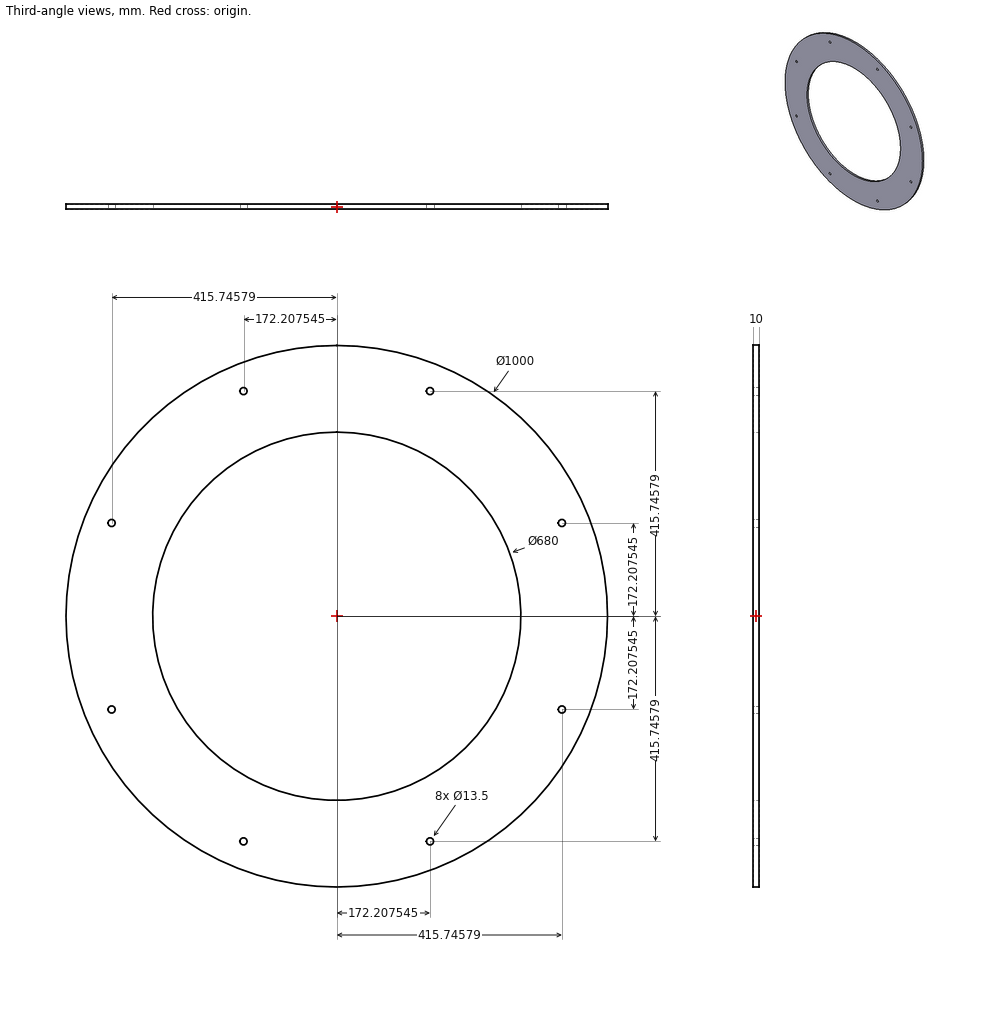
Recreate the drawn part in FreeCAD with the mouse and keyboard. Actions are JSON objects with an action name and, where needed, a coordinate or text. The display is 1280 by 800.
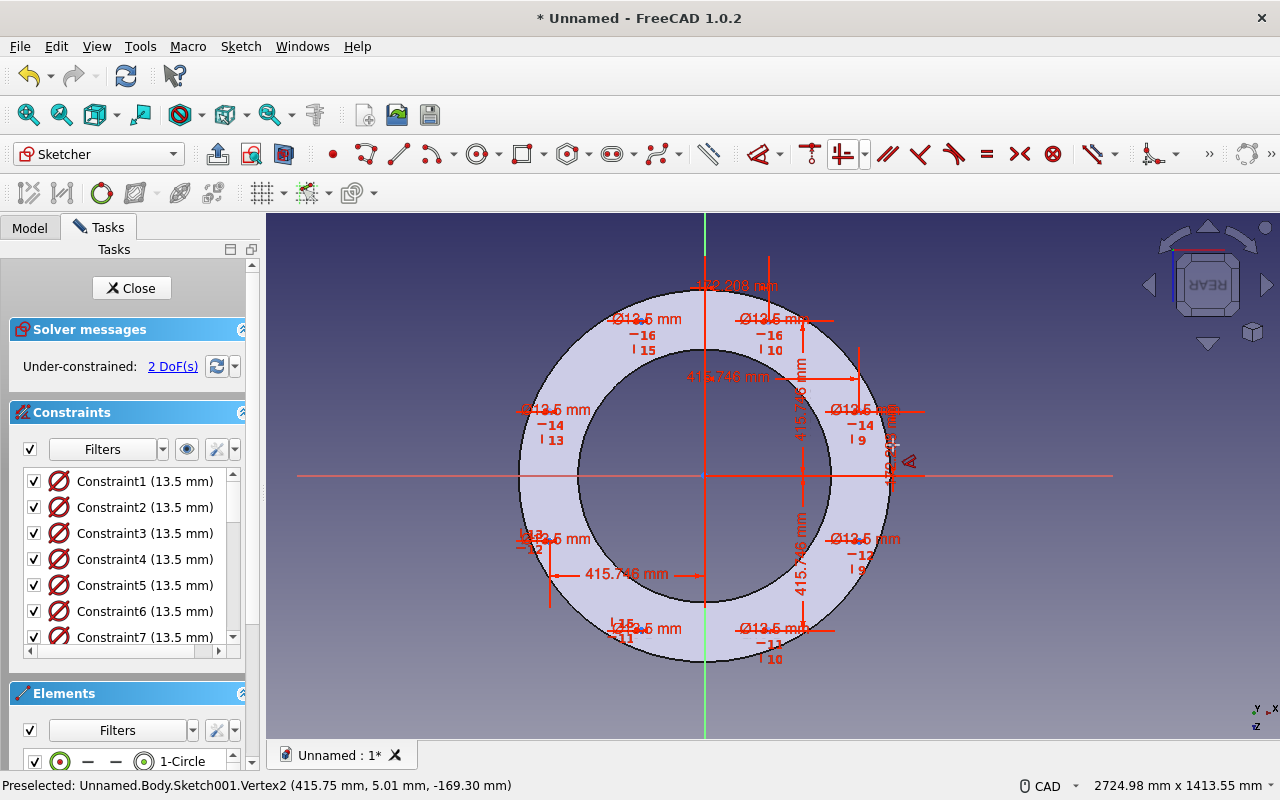
{"action": "left_click", "coordinate": [859, 541]}
{"action": "left_click", "coordinate": [893, 509]}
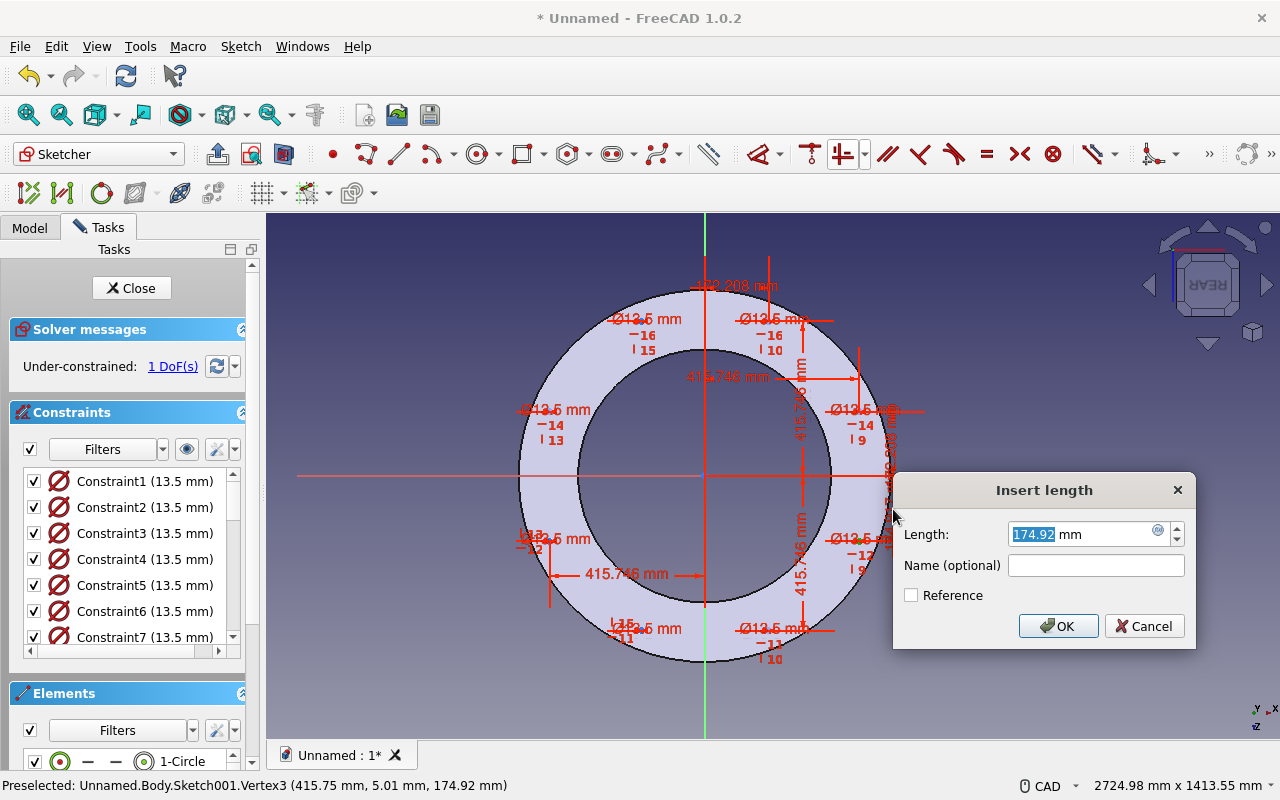
{"action": "type", "text": "172.207545"}
{"action": "key", "text": "Return"}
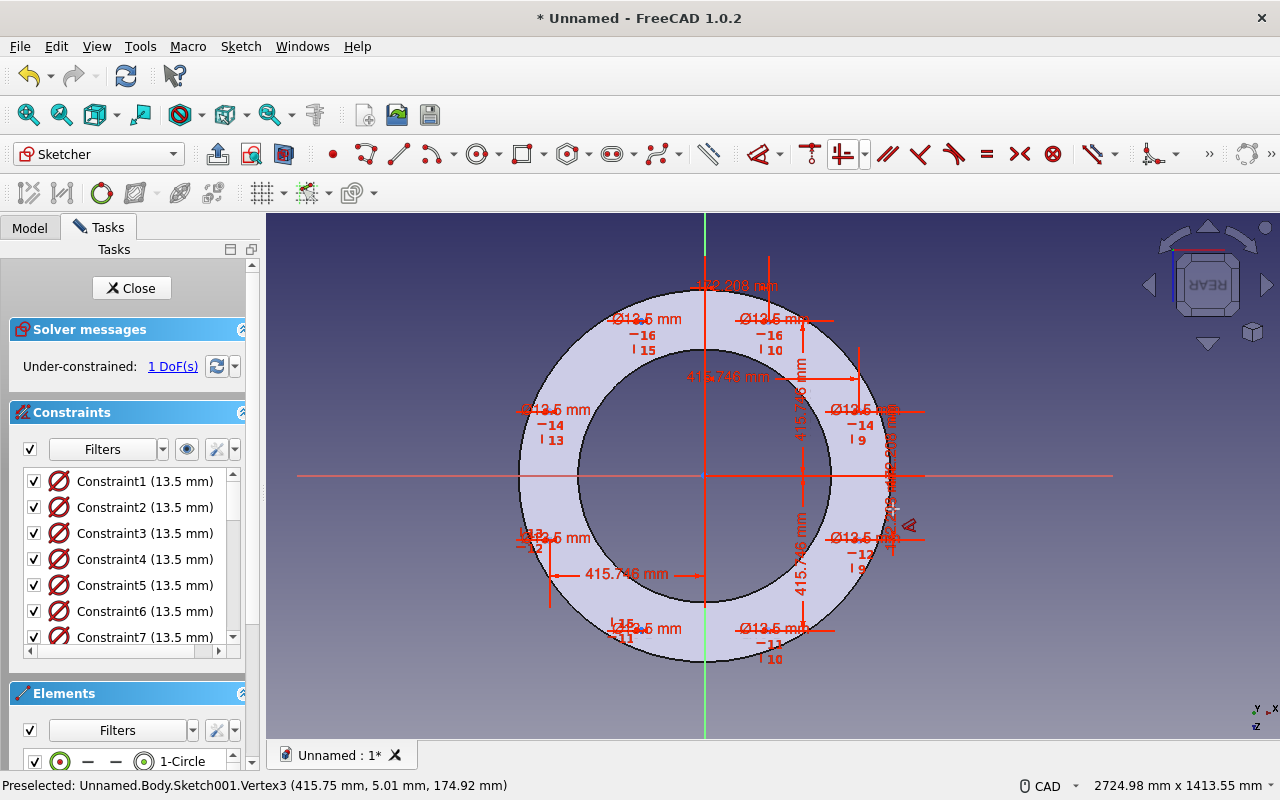
{"action": "left_click", "coordinate": [641, 631]}
{"action": "left_click", "coordinate": [673, 665]}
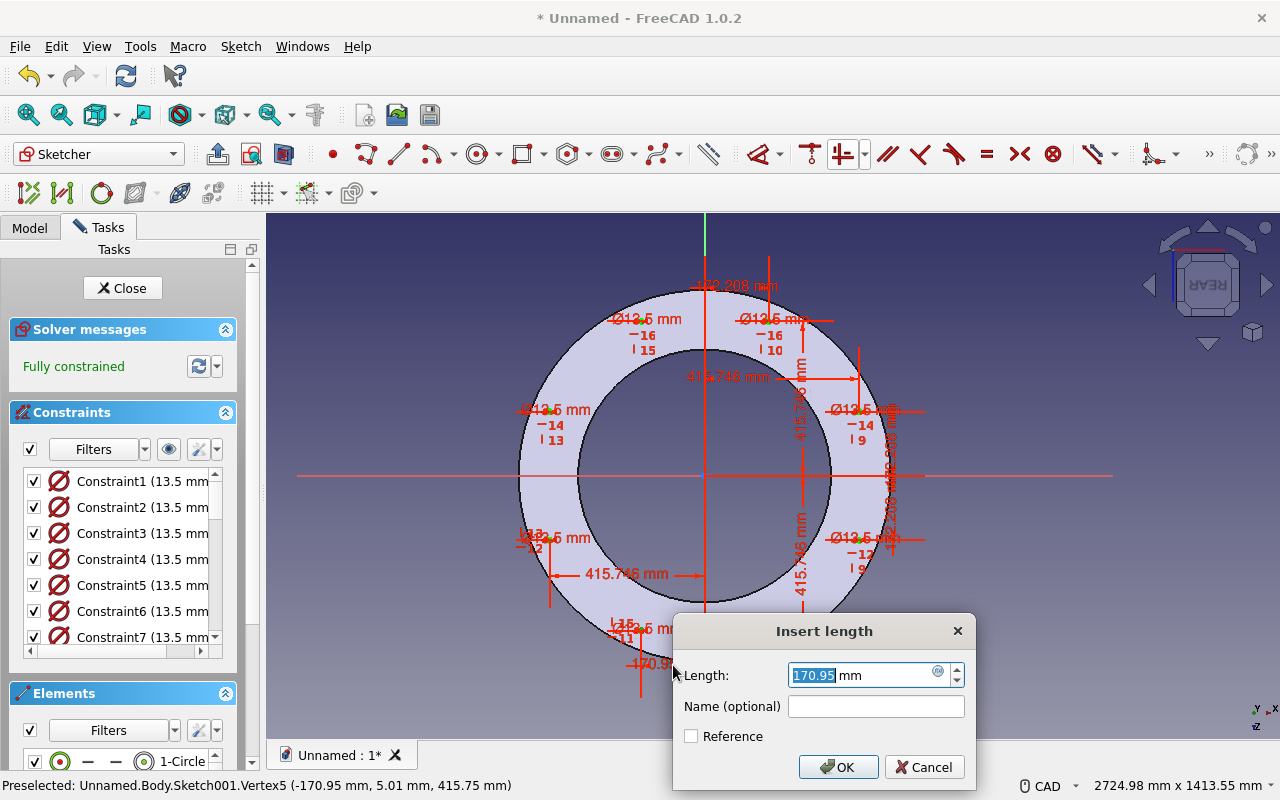
{"action": "type", "text": "172.207545"}
{"action": "key", "text": "Return"}
{"action": "key", "text": "Escape"}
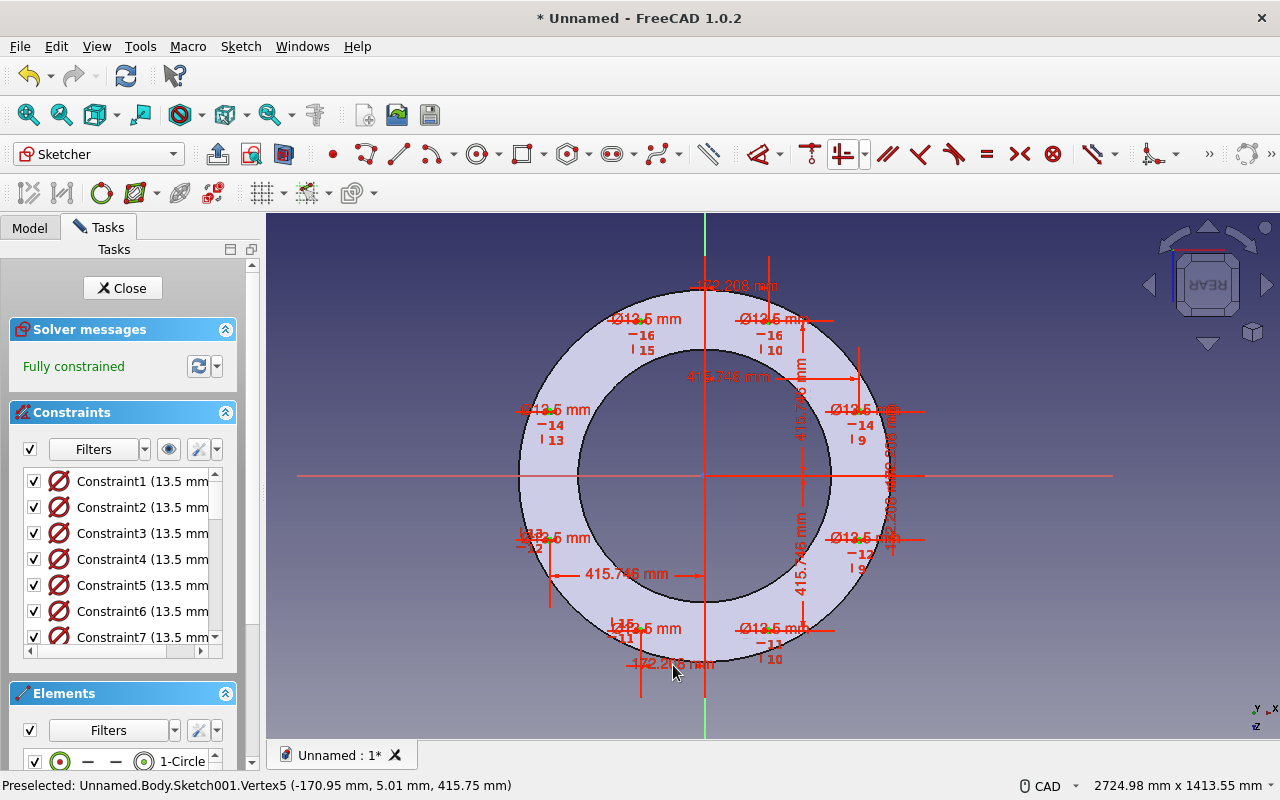
{"action": "left_click", "coordinate": [123, 288]}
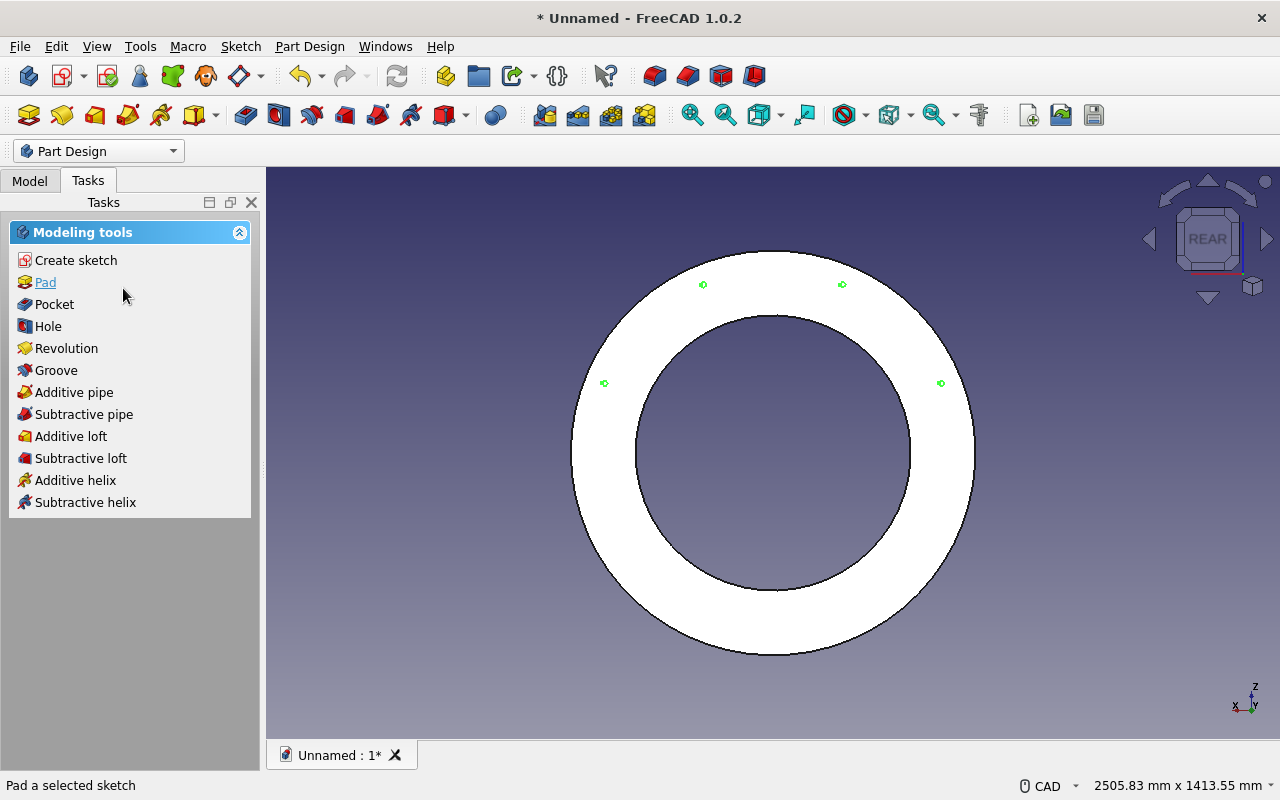
{"action": "left_click", "coordinate": [246, 116]}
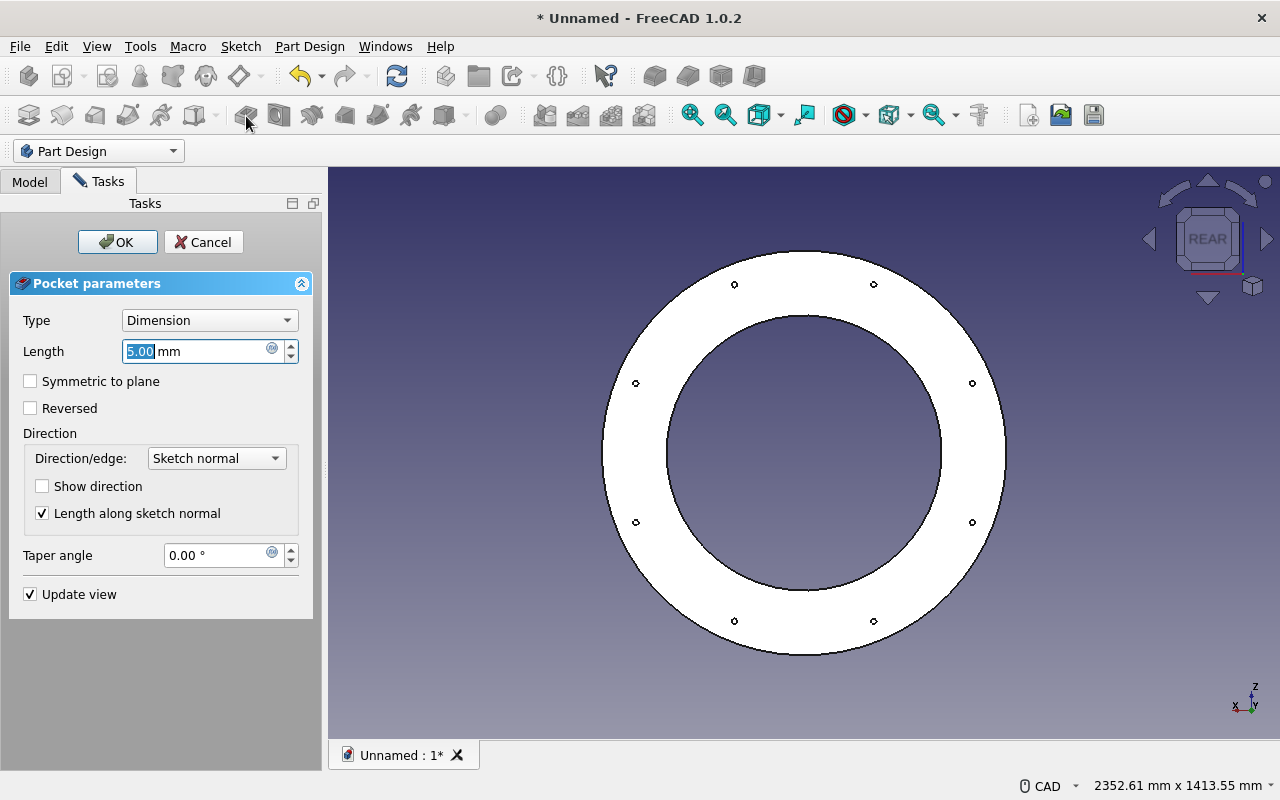
{"action": "left_click", "coordinate": [210, 320]}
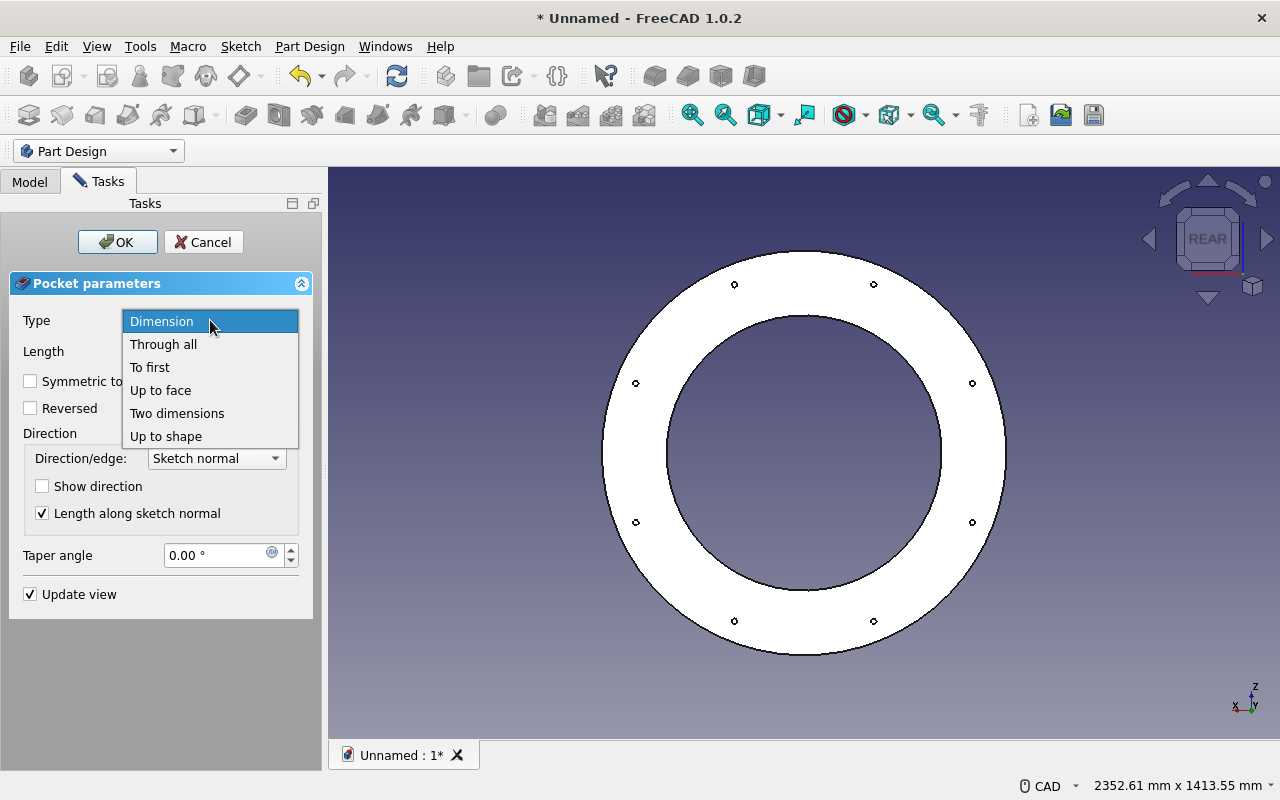
{"action": "left_click", "coordinate": [208, 344]}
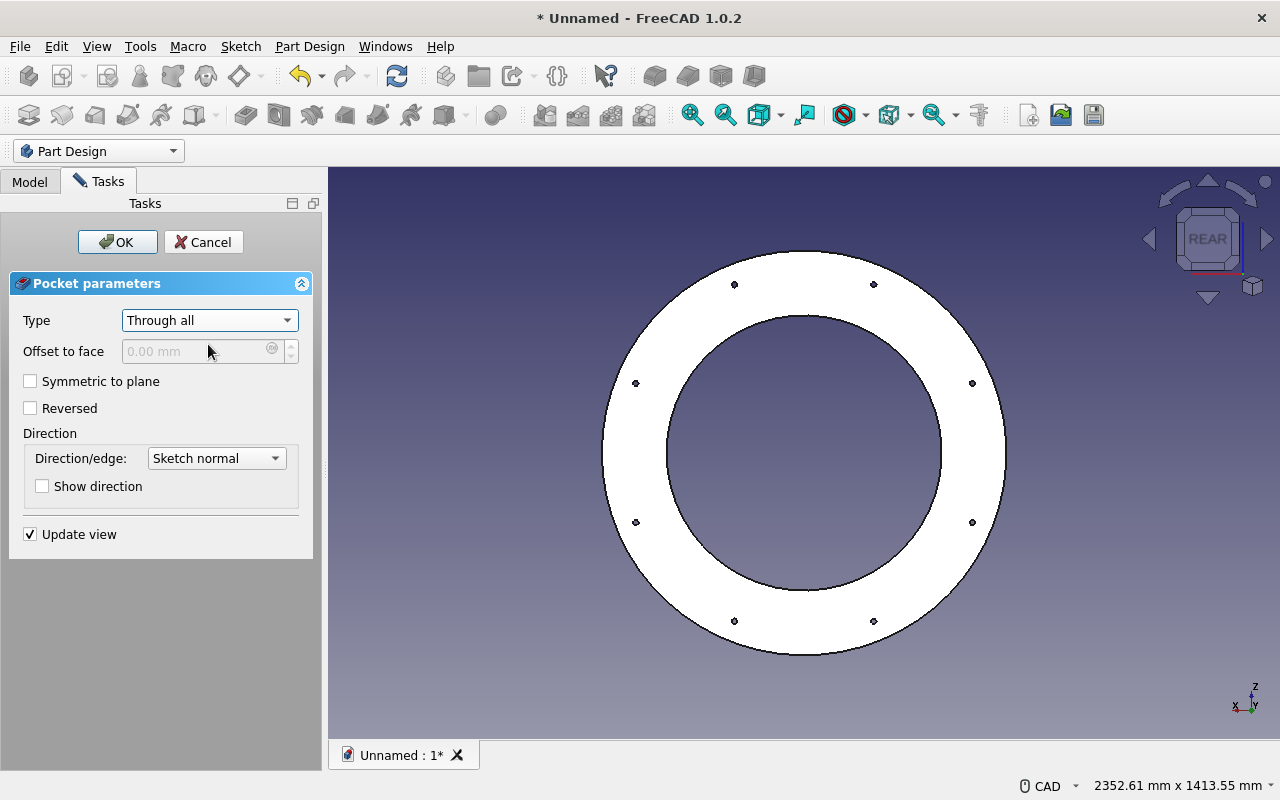
{"action": "left_click", "coordinate": [118, 242]}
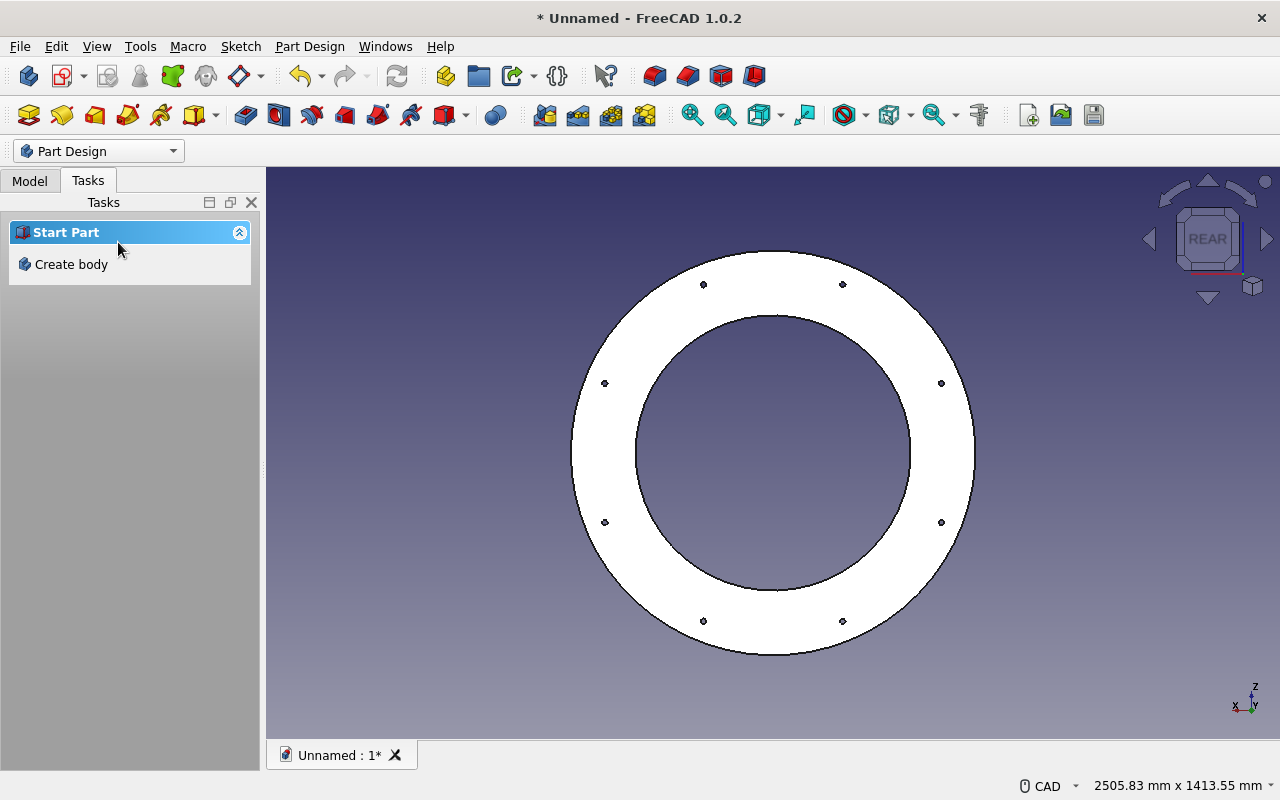
{"action": "key", "text": "0"}